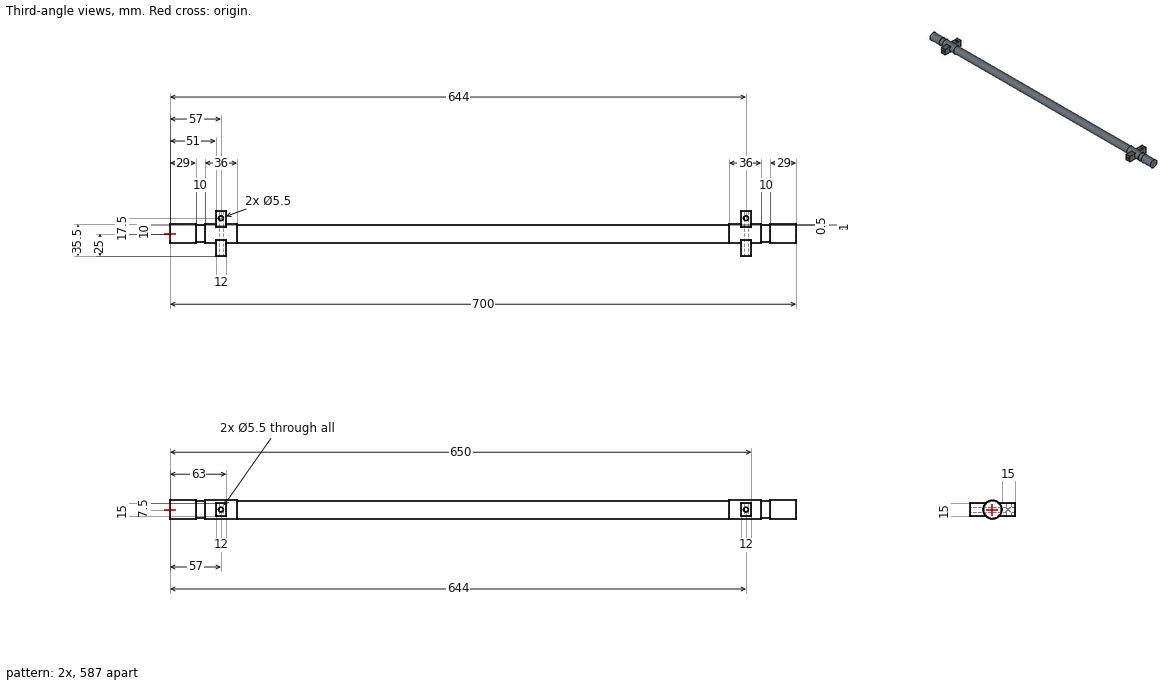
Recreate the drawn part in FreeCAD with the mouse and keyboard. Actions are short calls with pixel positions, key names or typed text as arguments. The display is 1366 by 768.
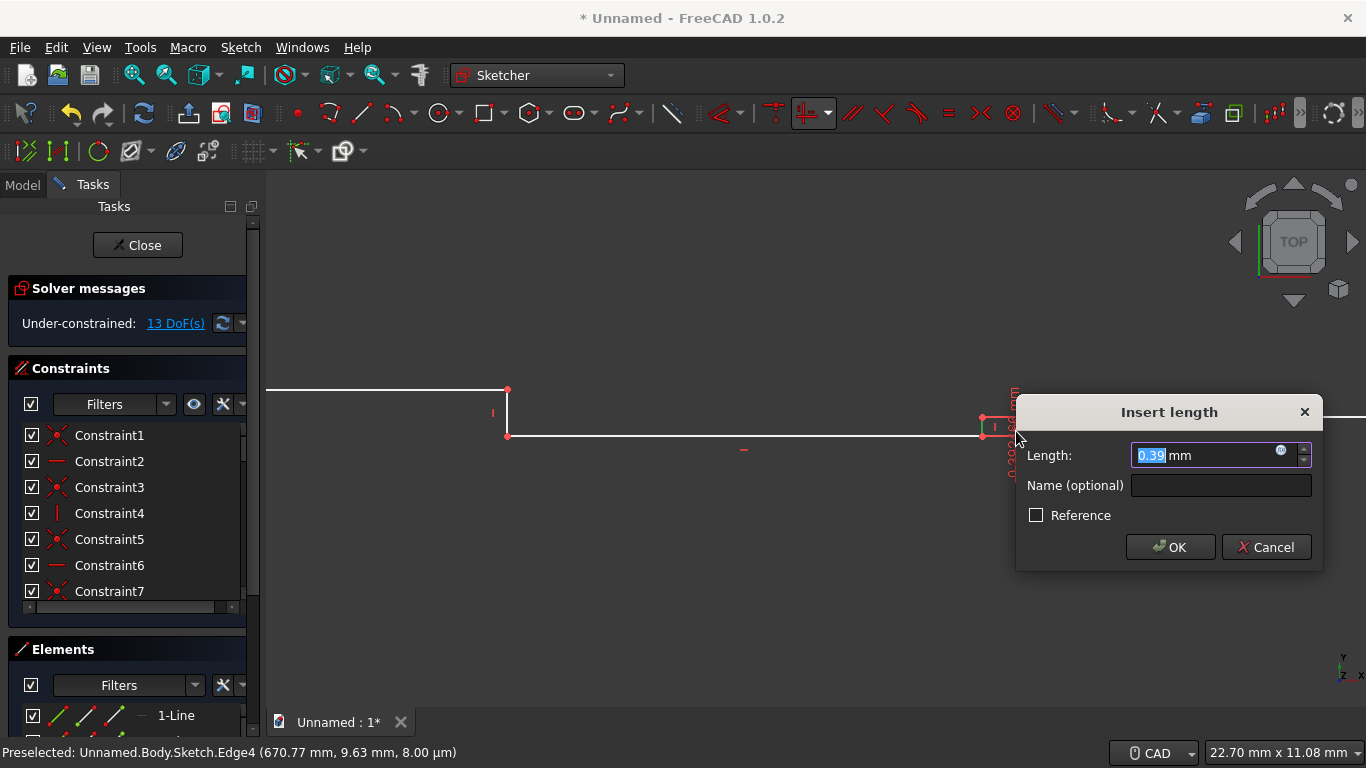
text(1)
key(Return)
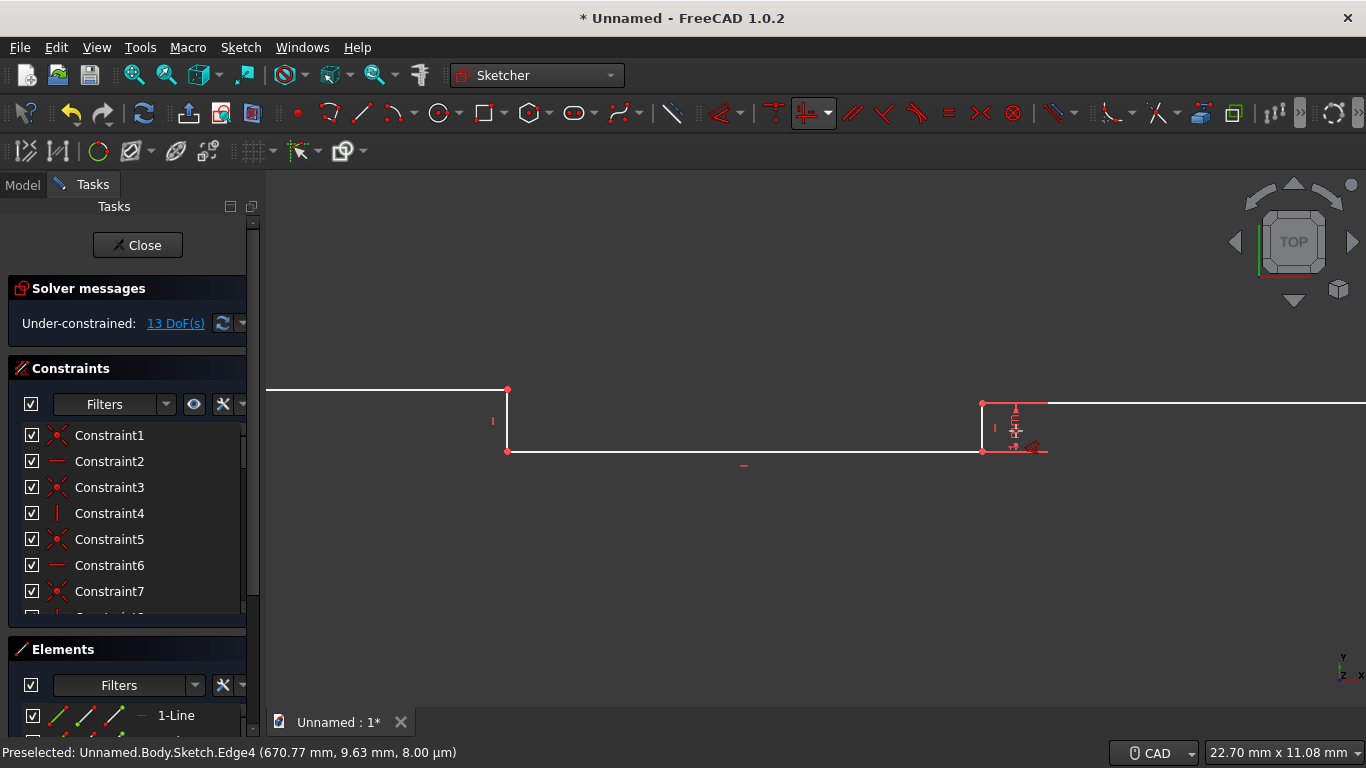
click(507, 433)
click(541, 421)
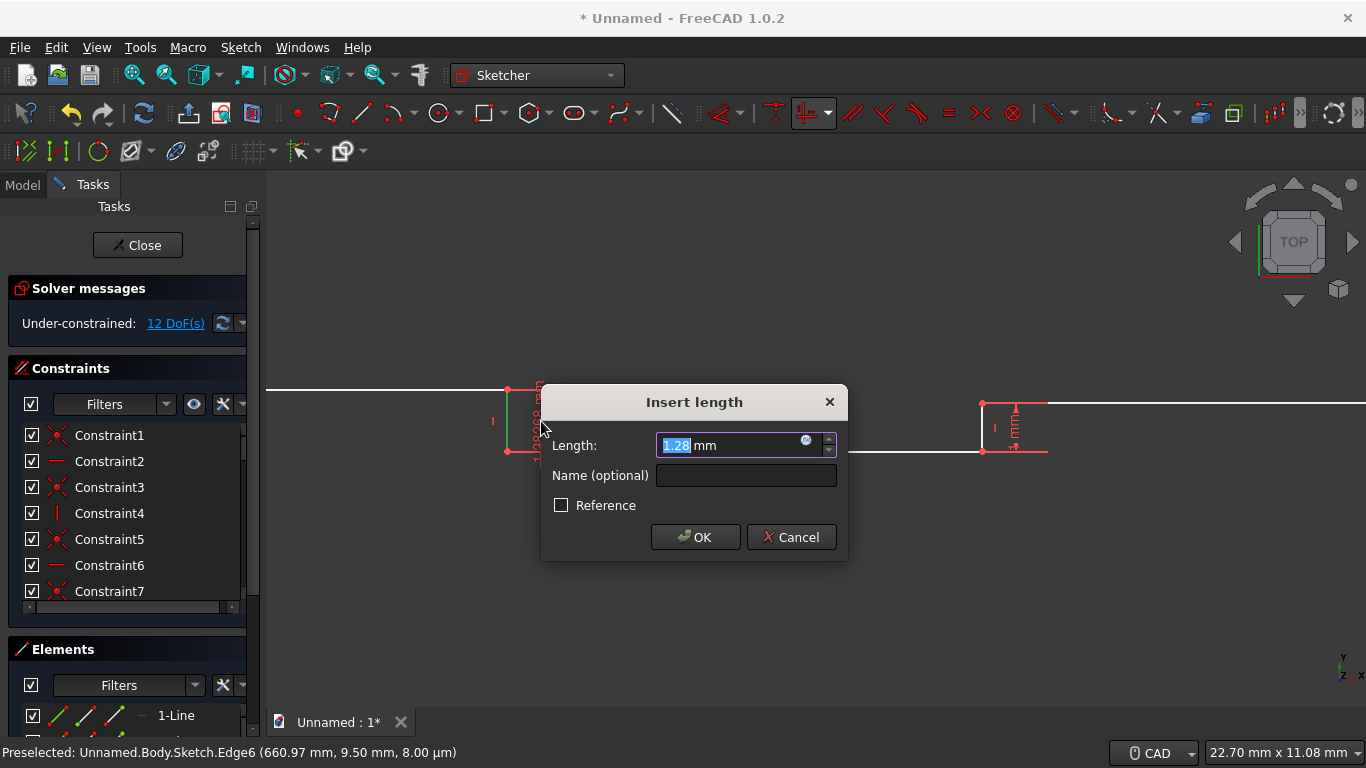
text(1)
key(Return)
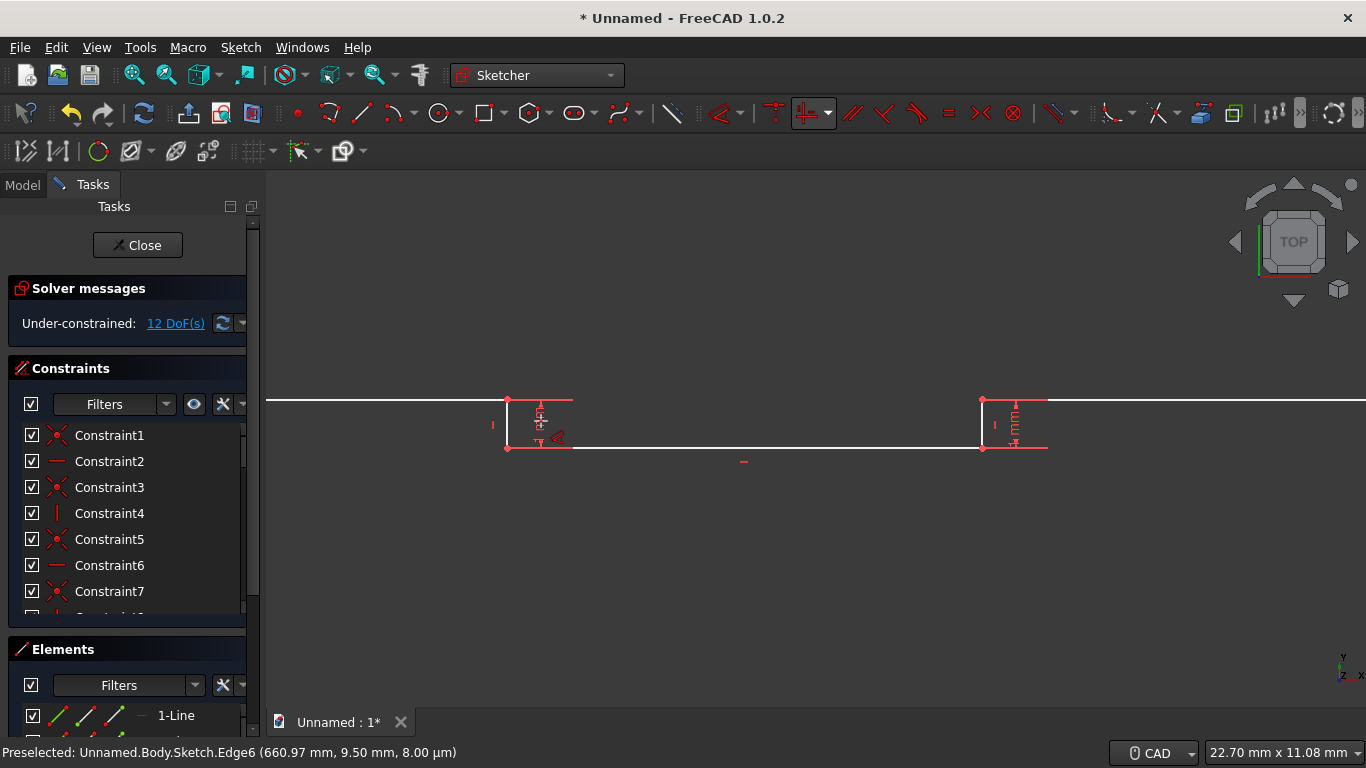
scroll(748, 438, down, 15)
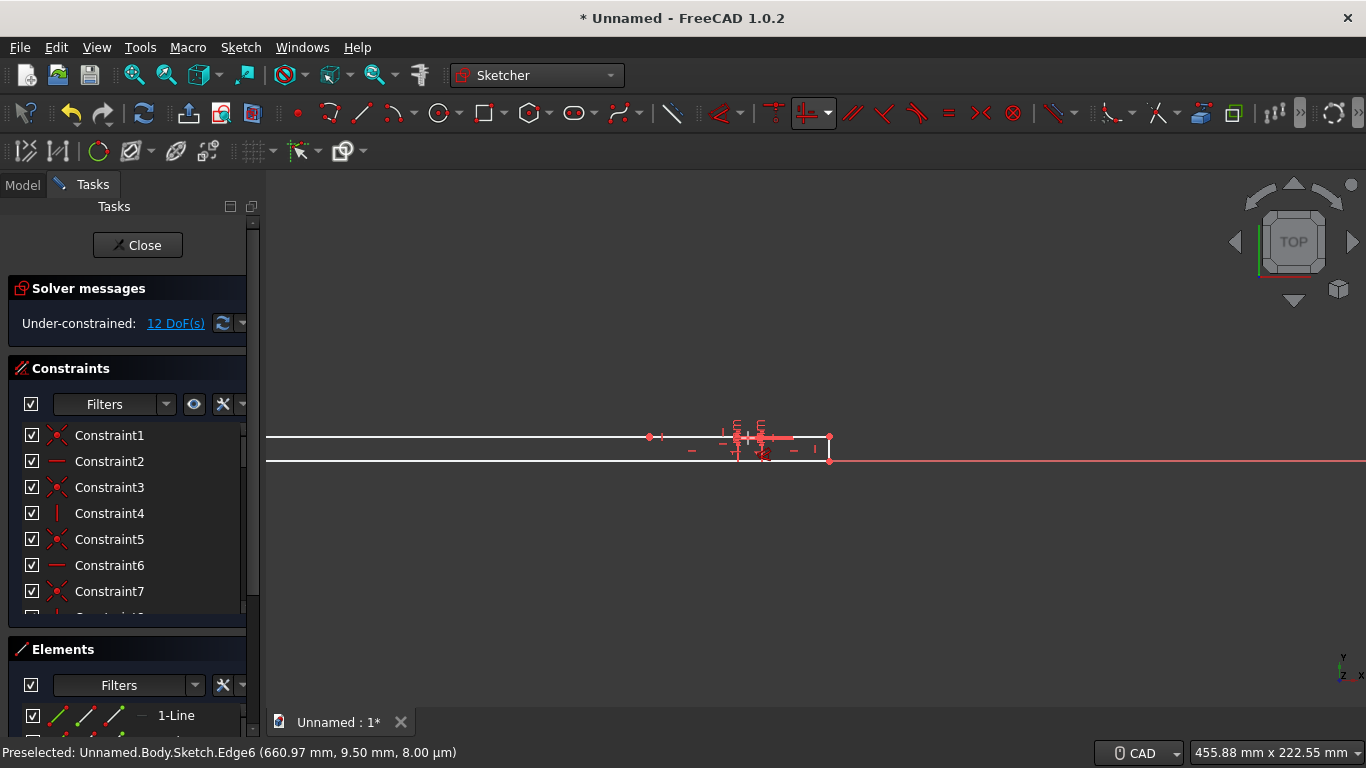
scroll(1191, 433, down, 5)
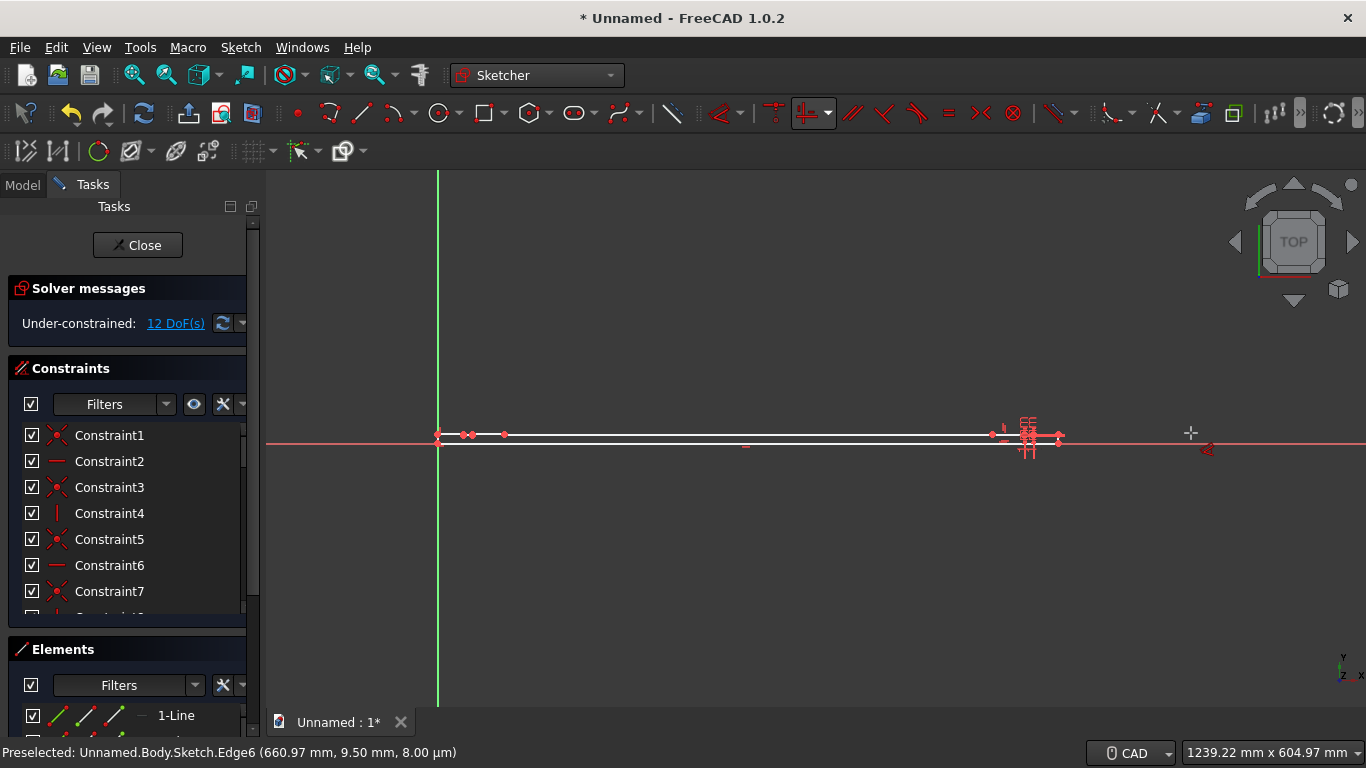
scroll(472, 435, up, 20)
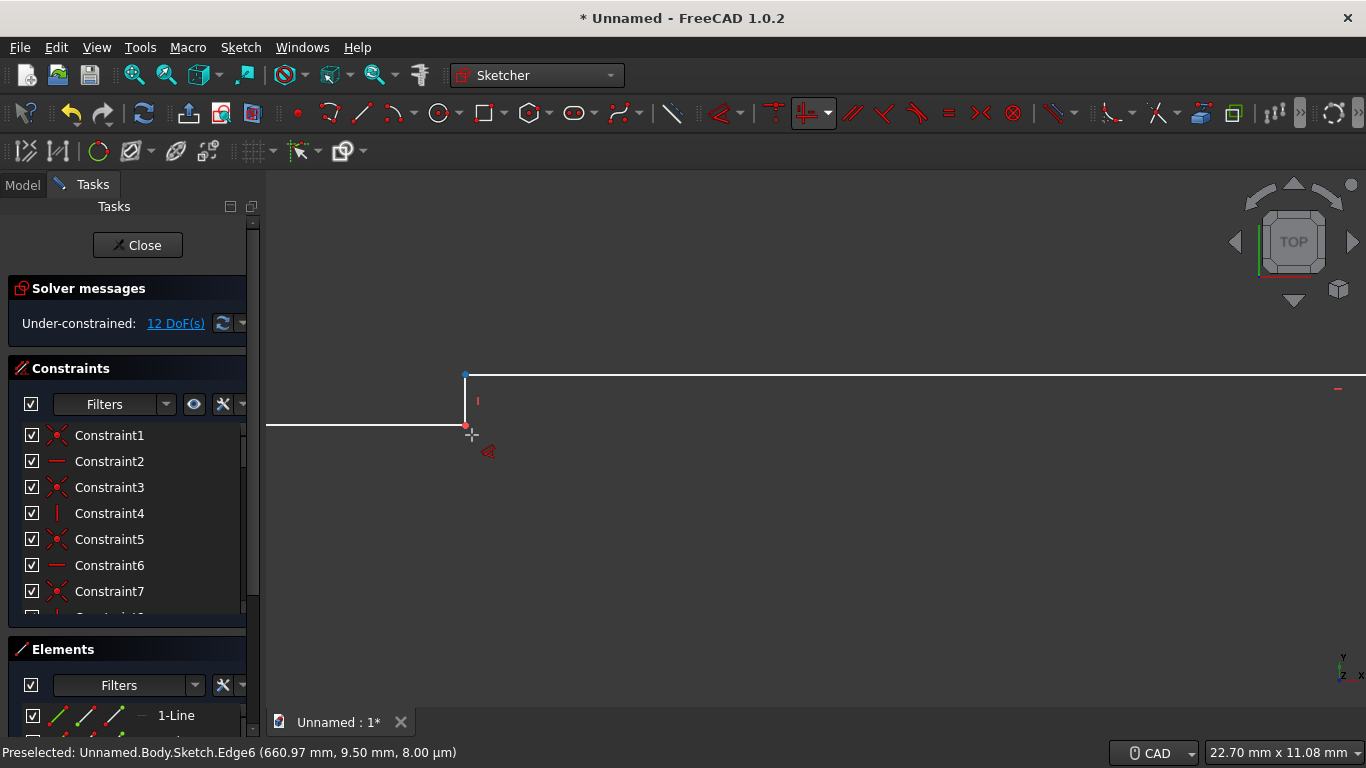
click(465, 390)
click(431, 400)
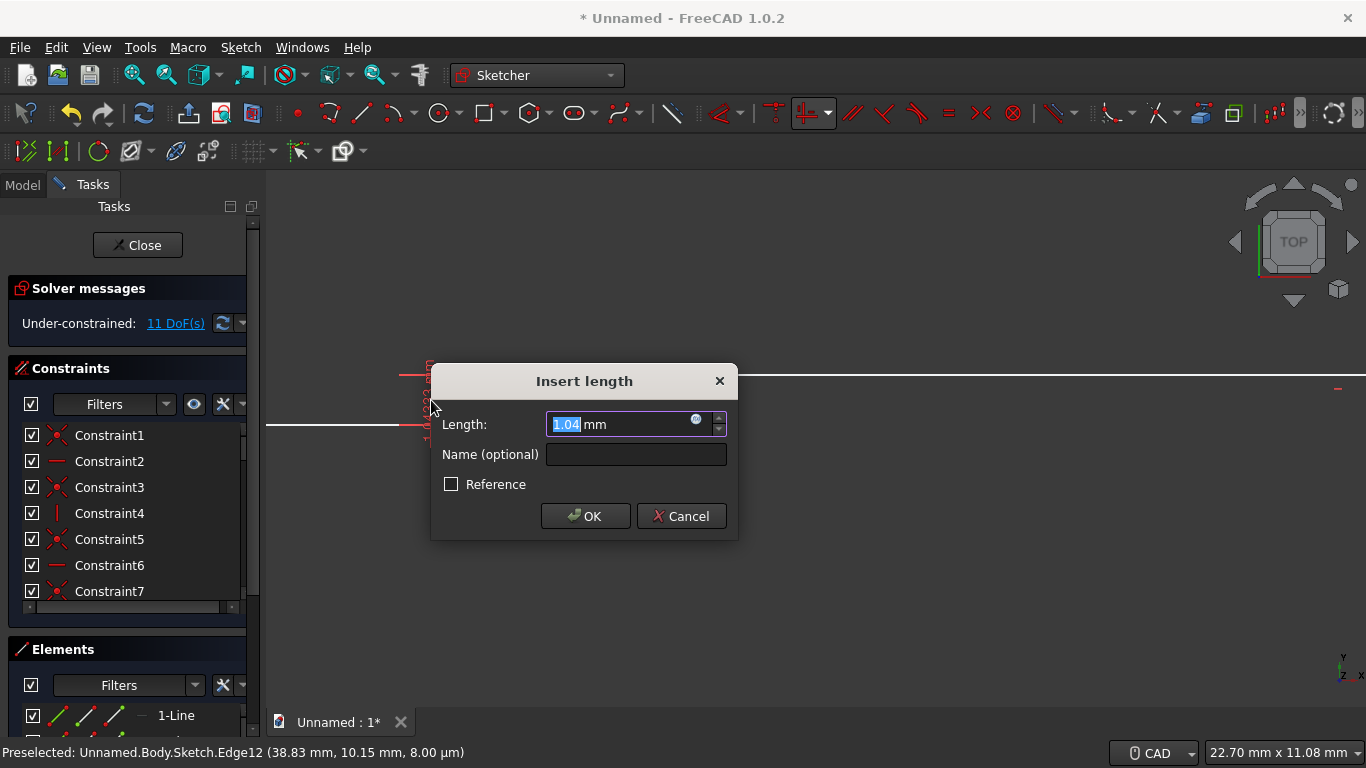
text(1)
key(Return)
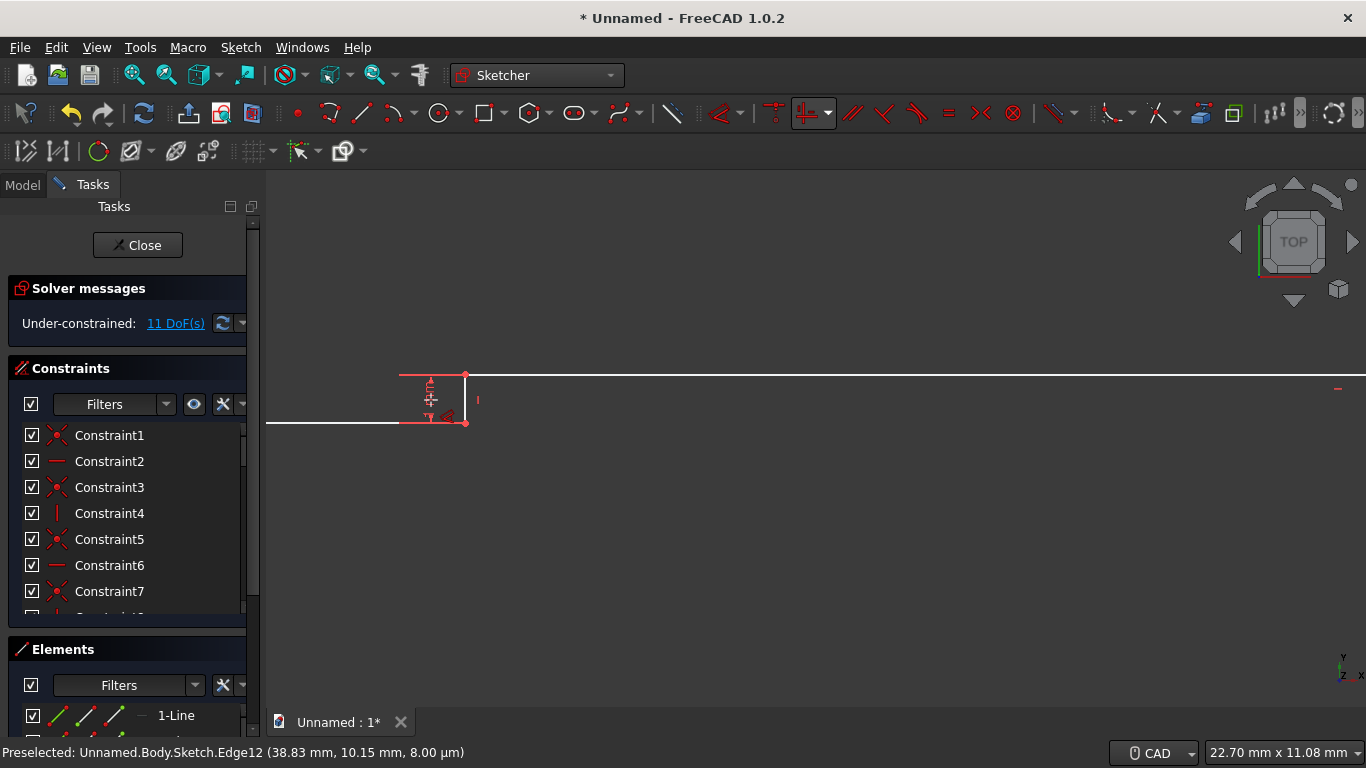
scroll(748, 438, down, 15)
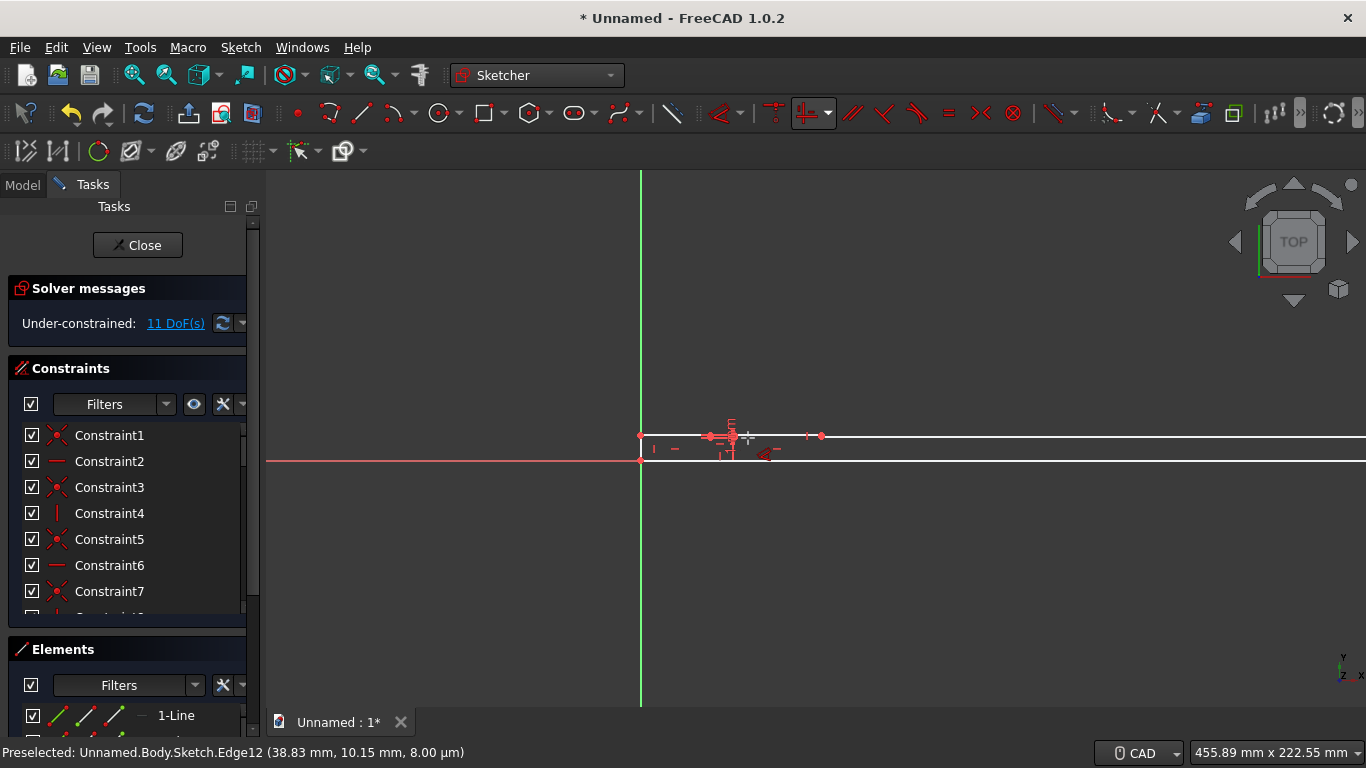
scroll(318, 433, down, 5)